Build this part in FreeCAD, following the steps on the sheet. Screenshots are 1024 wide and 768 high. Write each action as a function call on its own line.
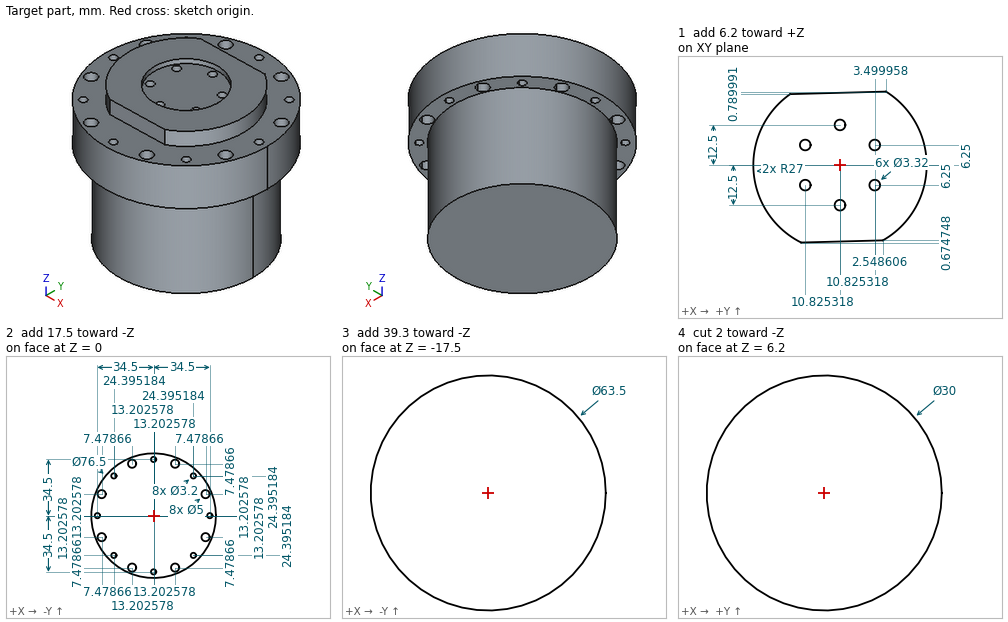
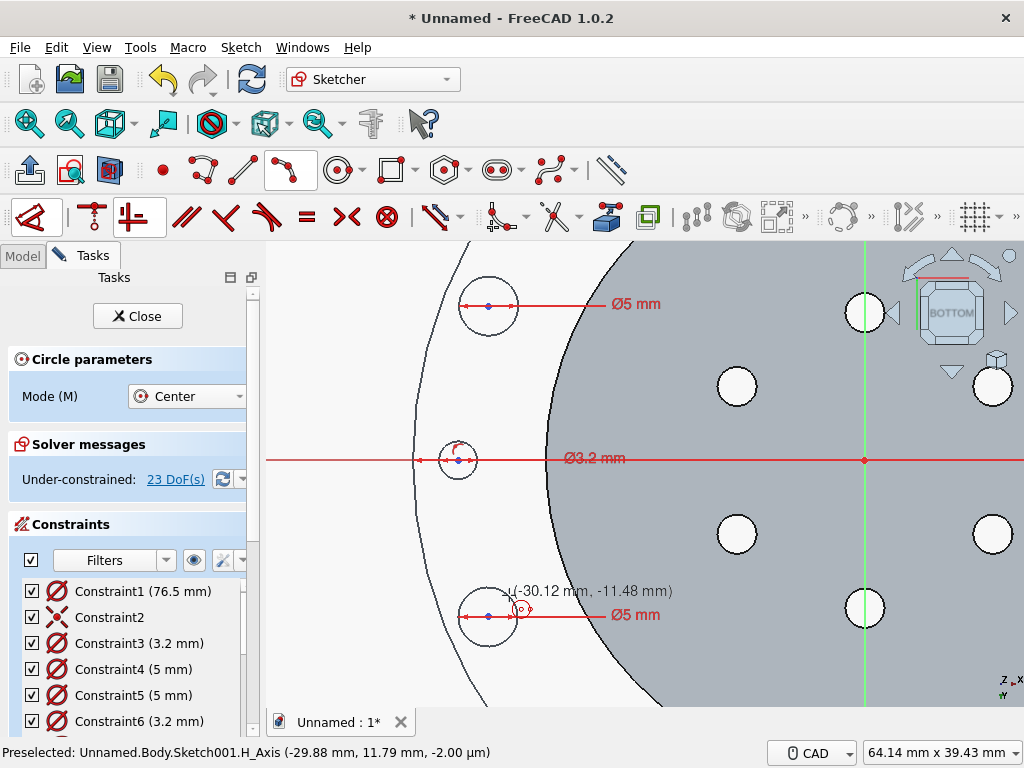
scroll(452, 480, down, 6)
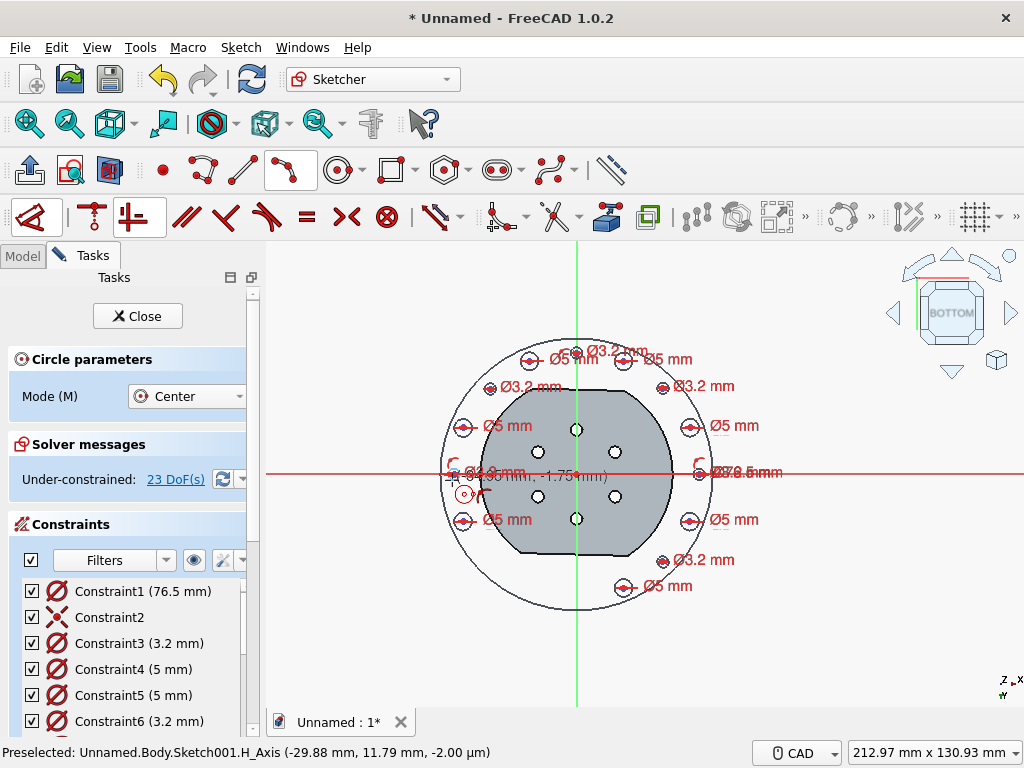
scroll(577, 597, up, 7)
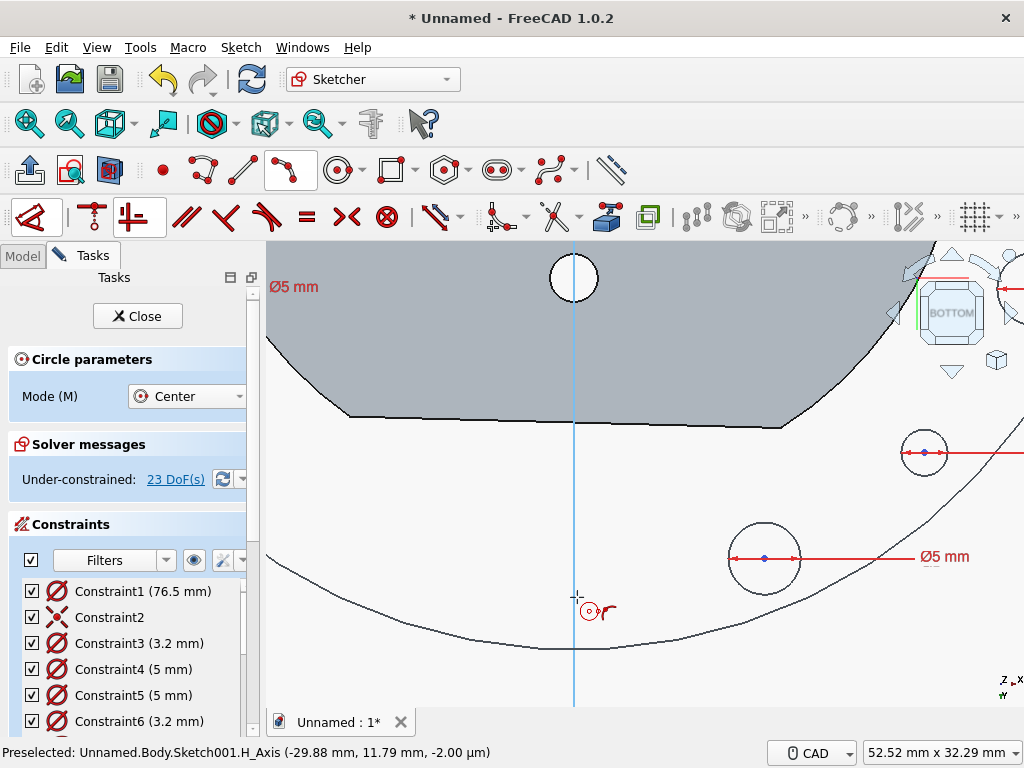
scroll(577, 597, down, 7)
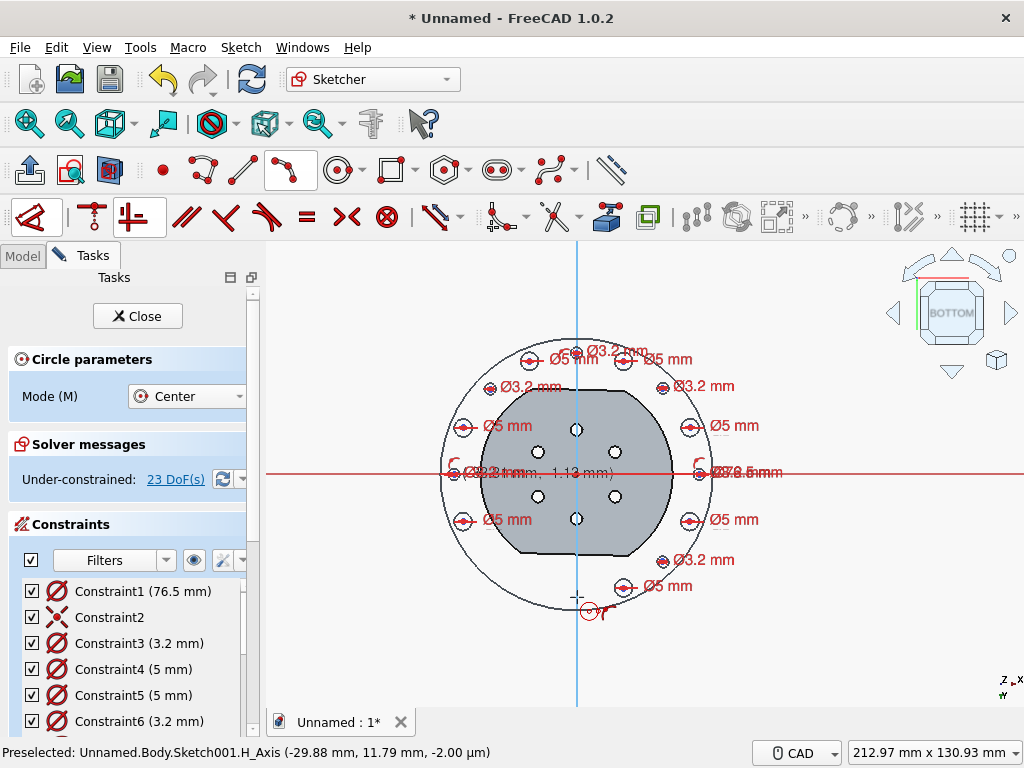
click(577, 597)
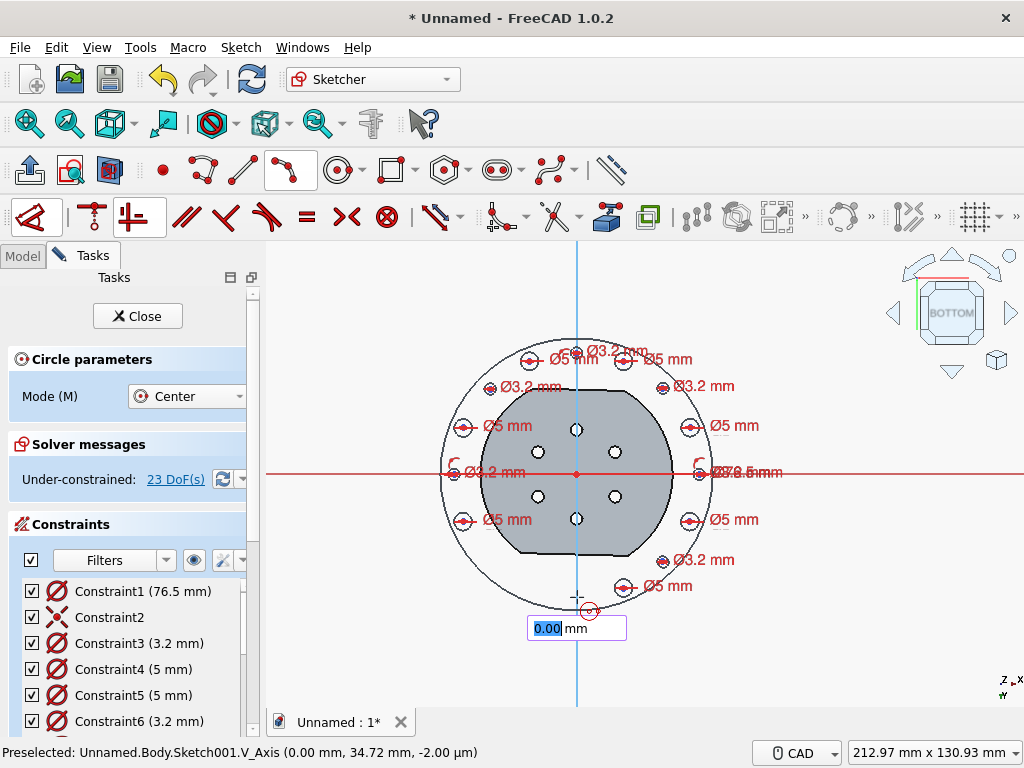
scroll(582, 595, up, 6)
move(581, 594)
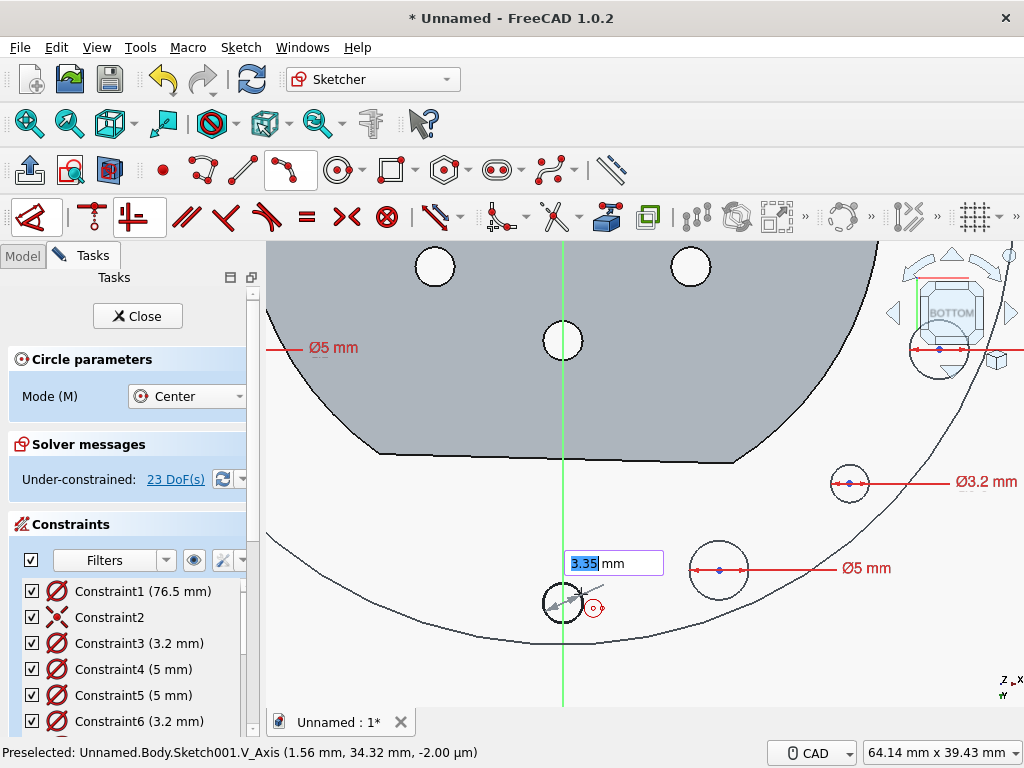
text(3.2)
key(Return)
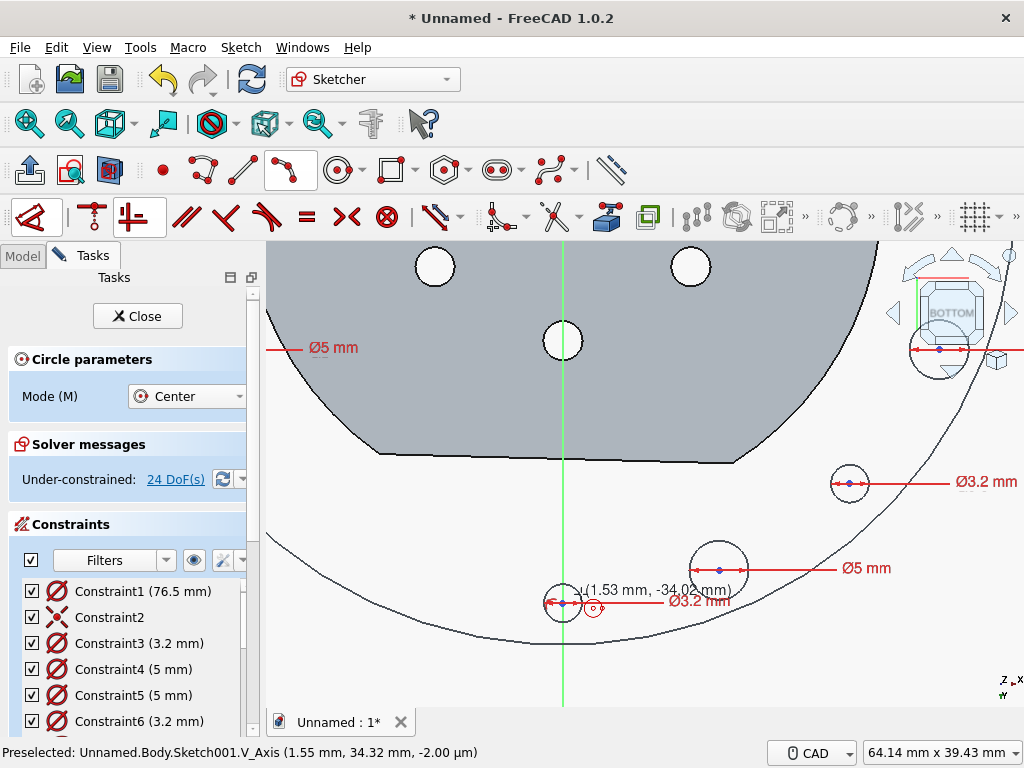
click(407, 570)
move(428, 549)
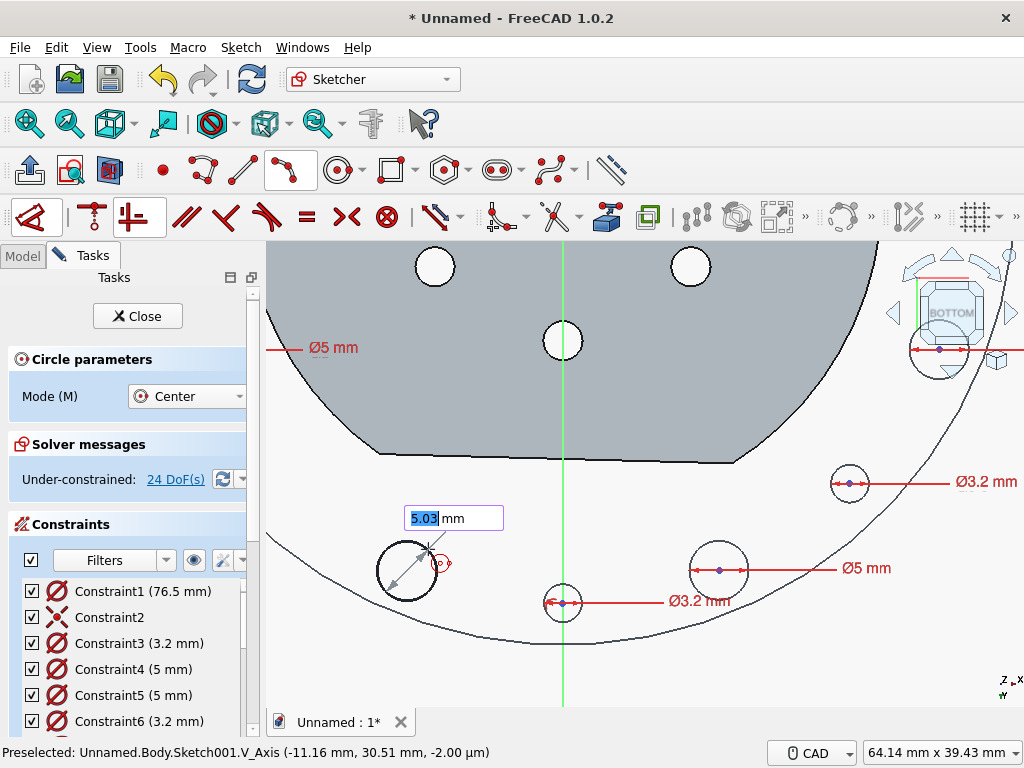
text(5)
key(Return)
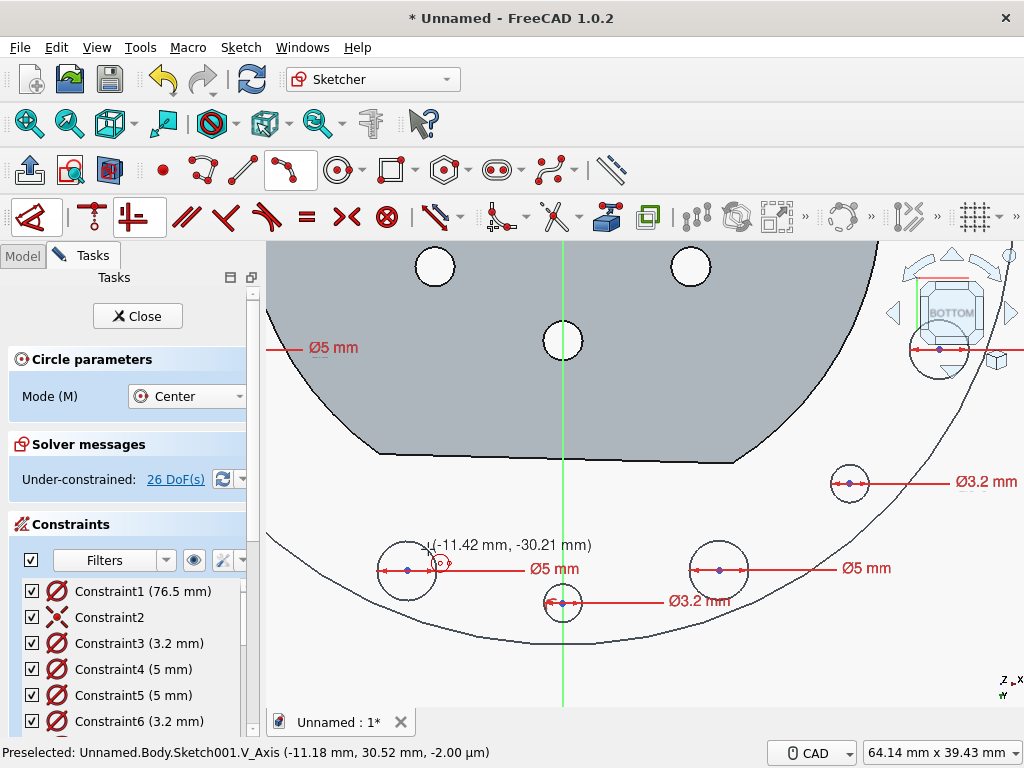
scroll(582, 595, down, 6)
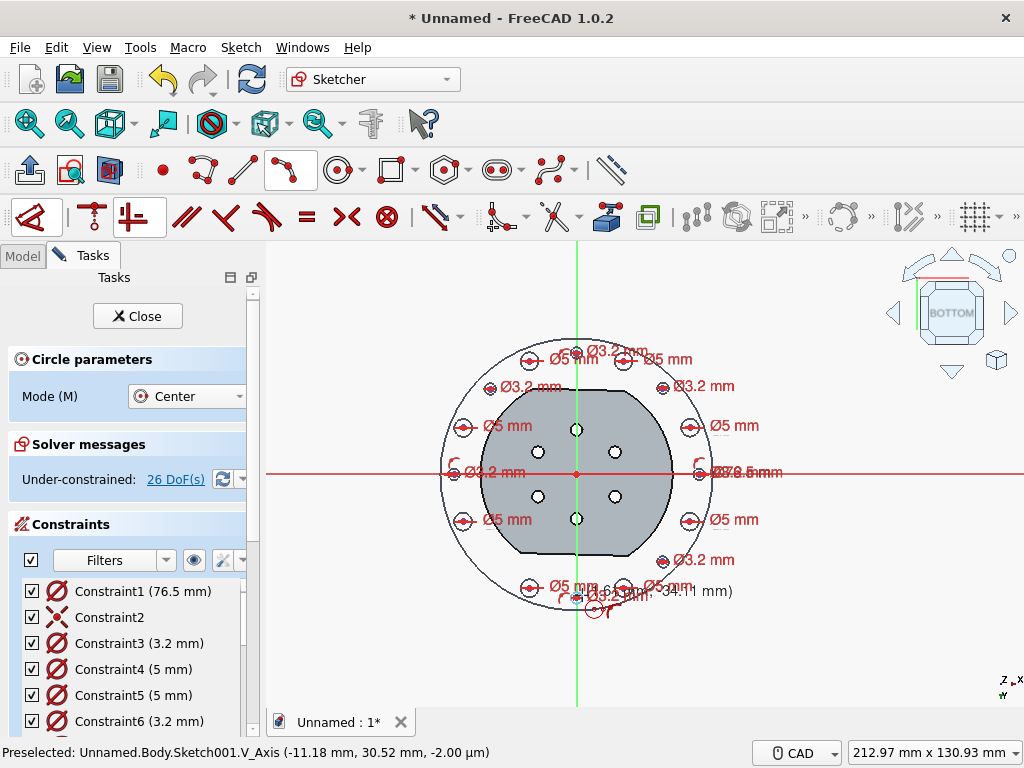
scroll(490, 561, up, 7)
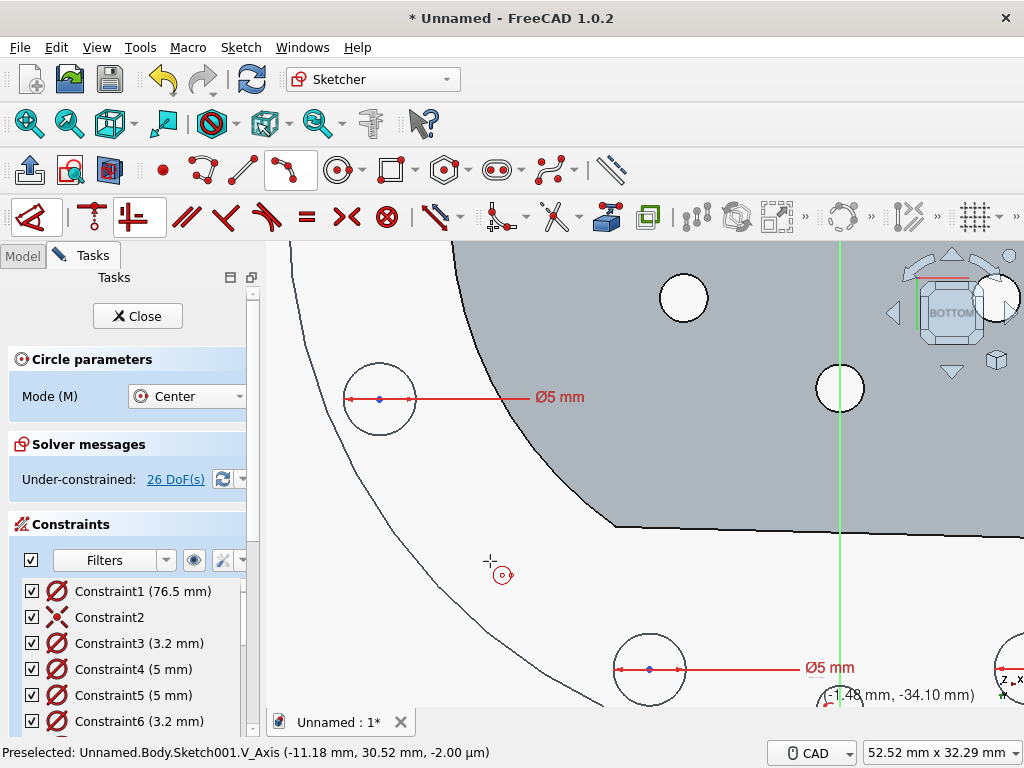
scroll(490, 561, down, 7)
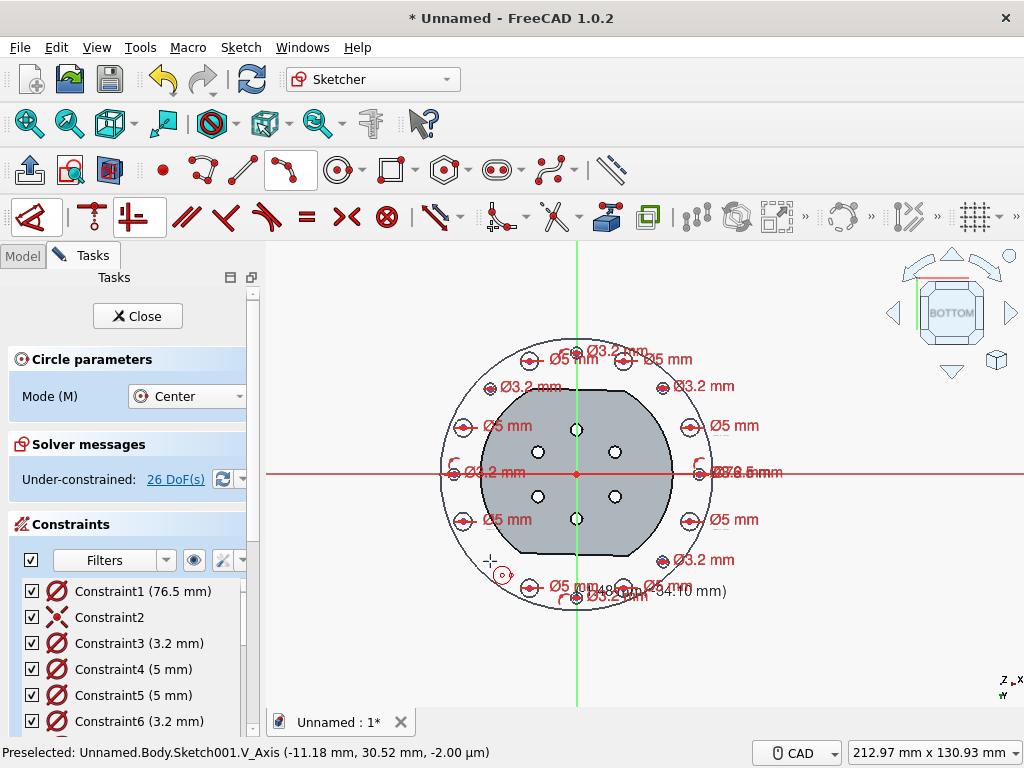
click(490, 561)
move(494, 557)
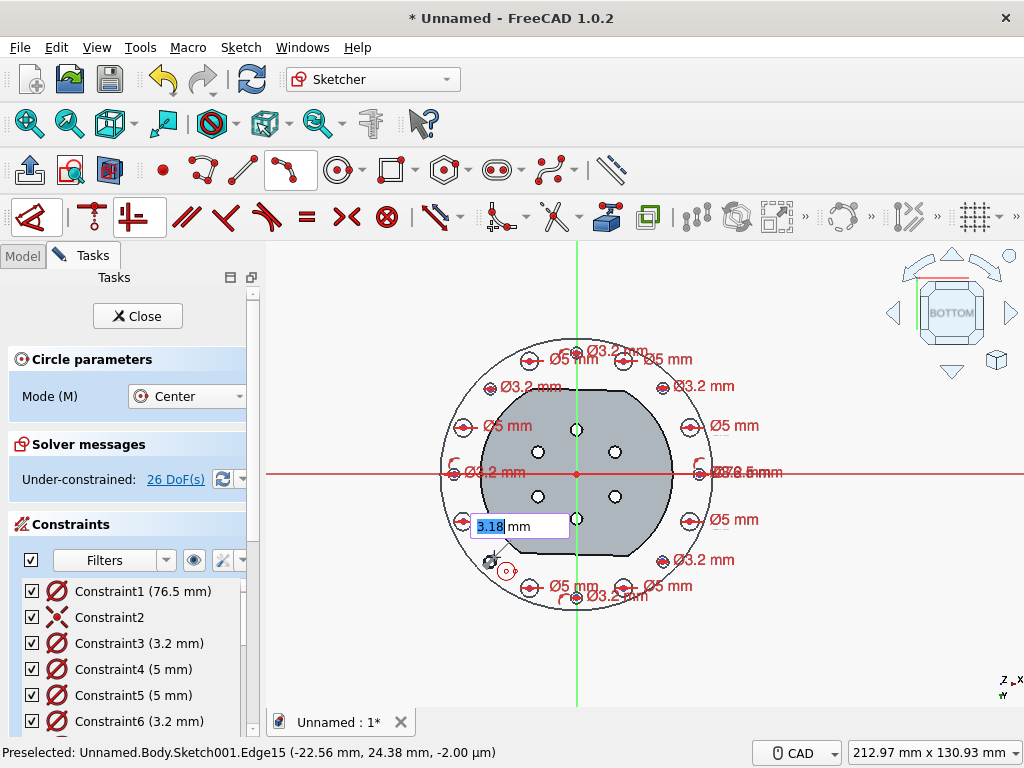
text(3.2)
key(Return)
key(Escape)